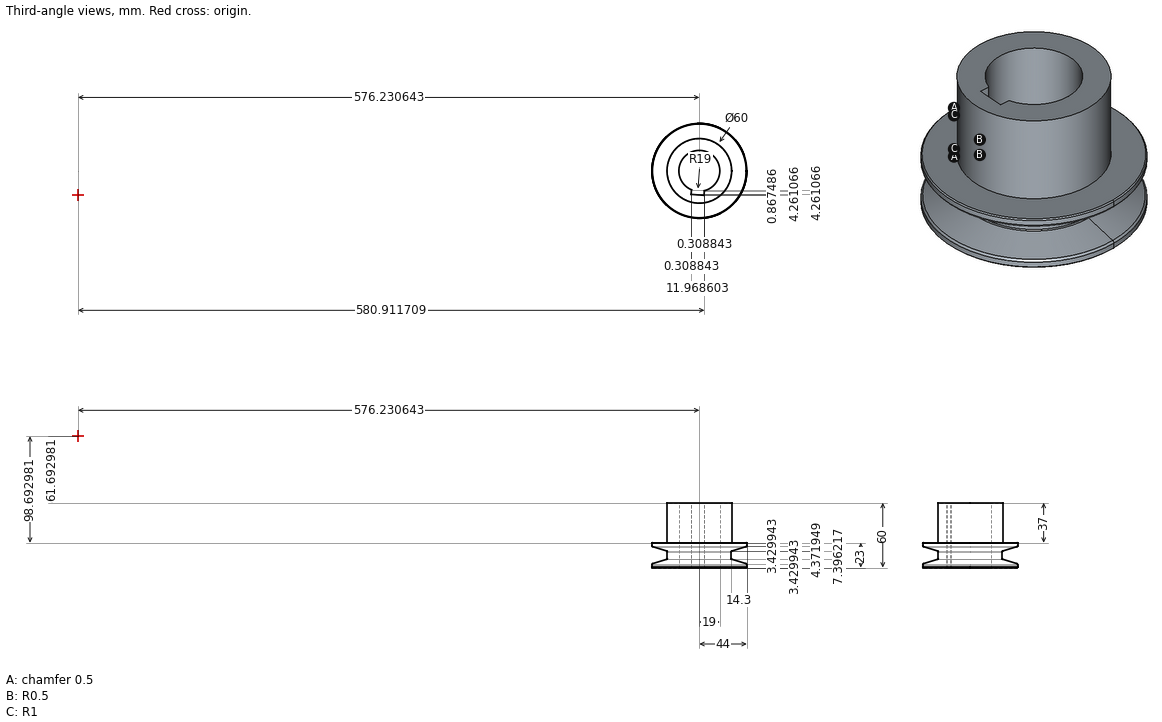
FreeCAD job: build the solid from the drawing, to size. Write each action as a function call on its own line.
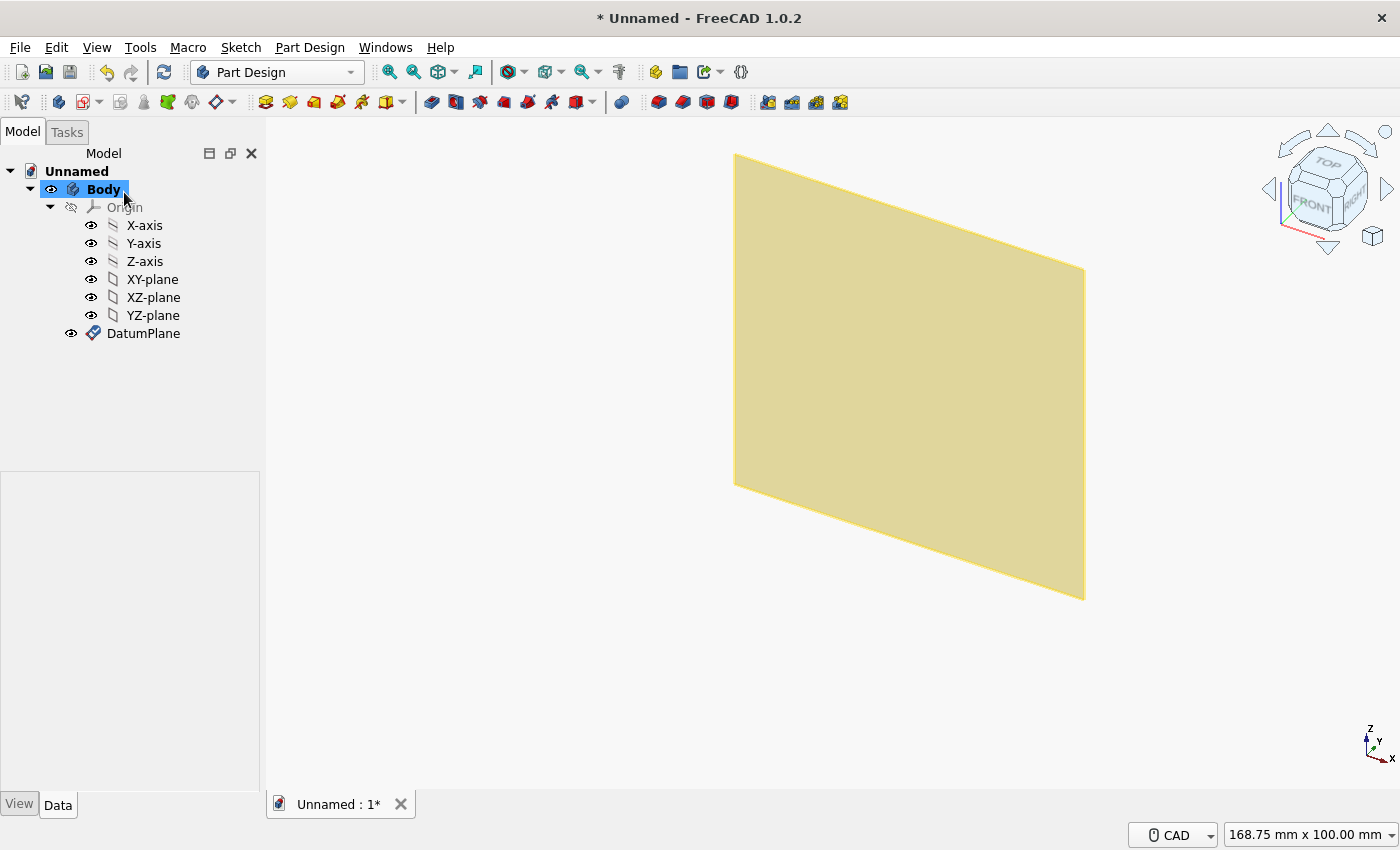
click(116, 333)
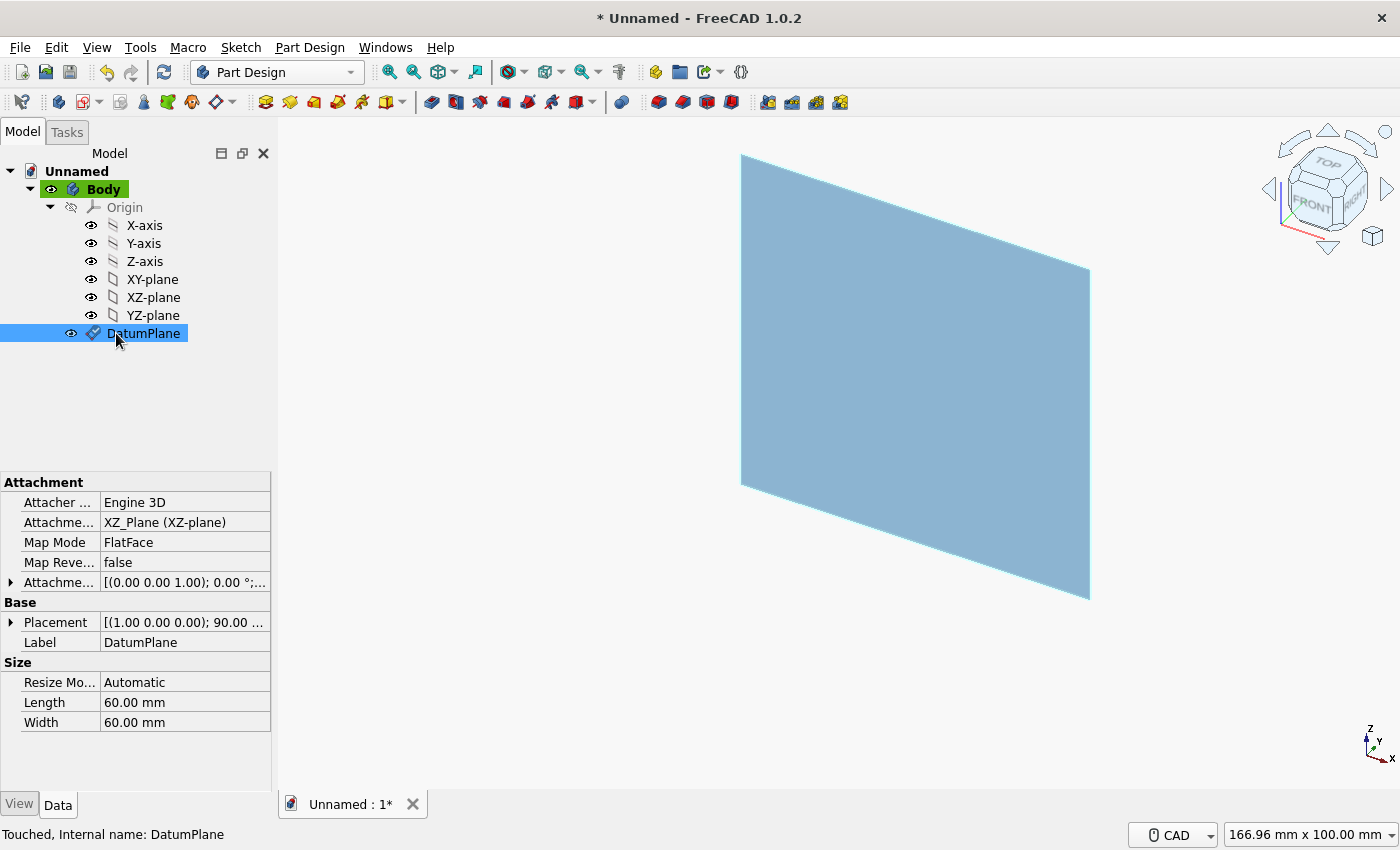
click(84, 102)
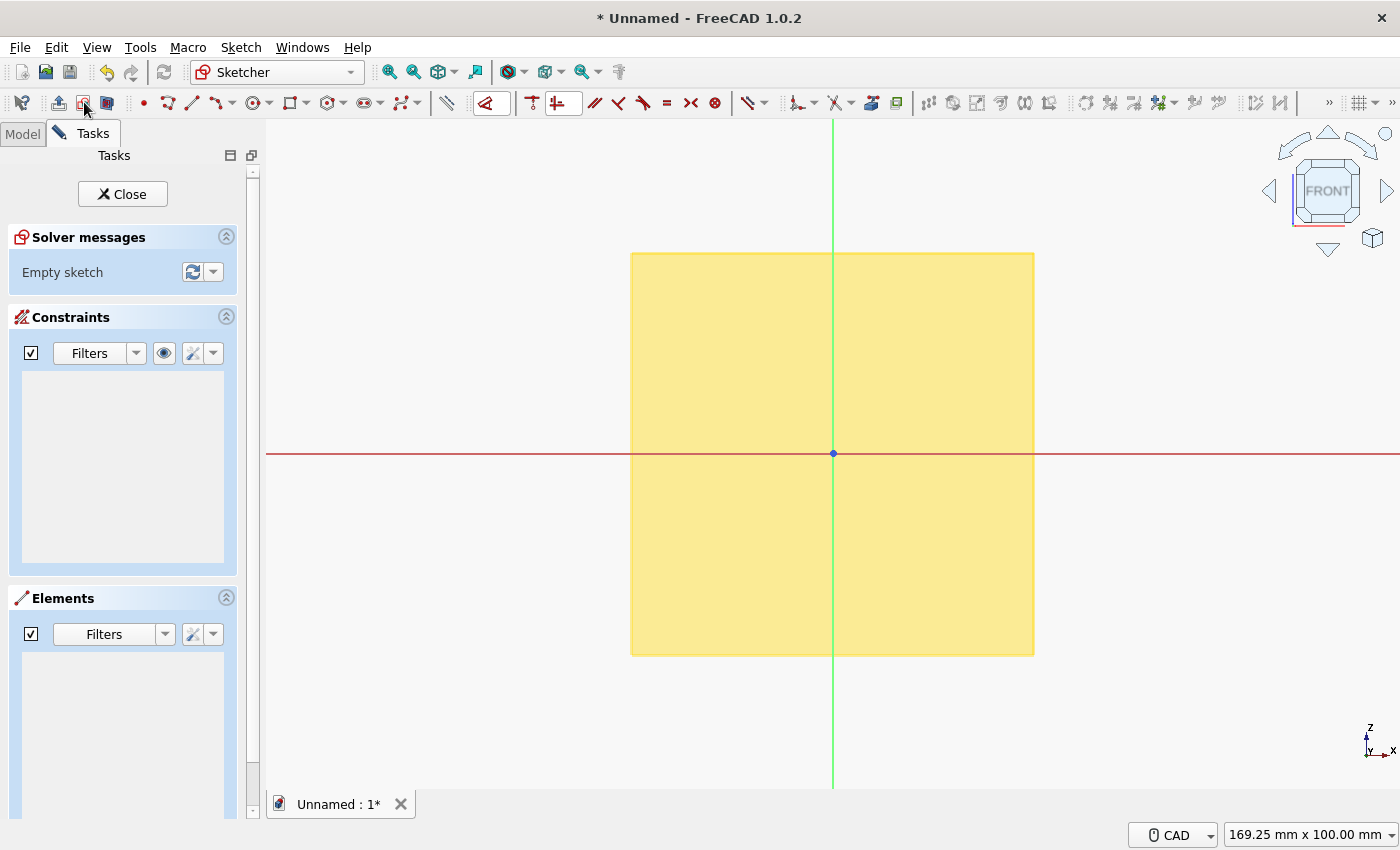
scroll(764, 454, down, 5)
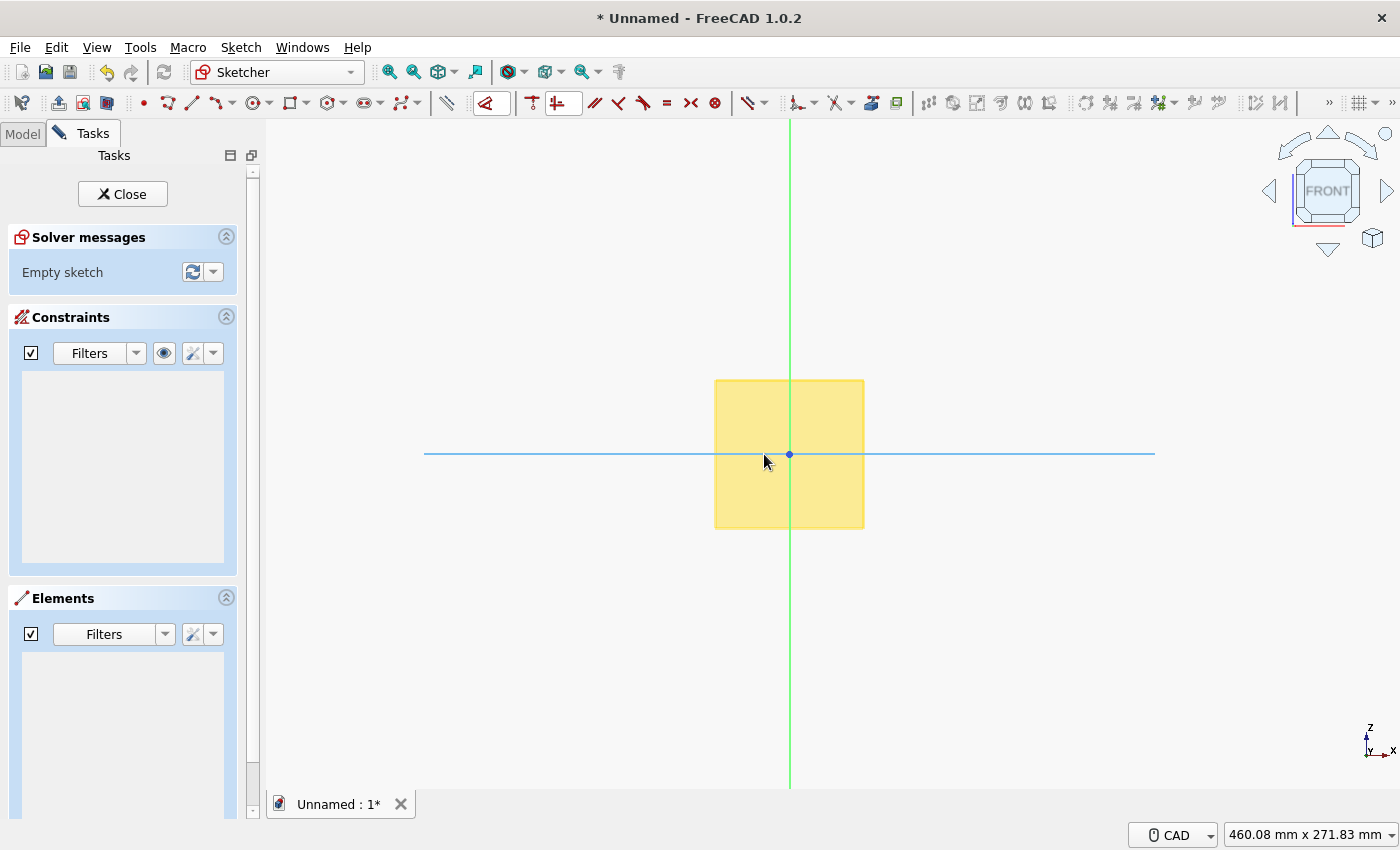
scroll(764, 454, down, 5)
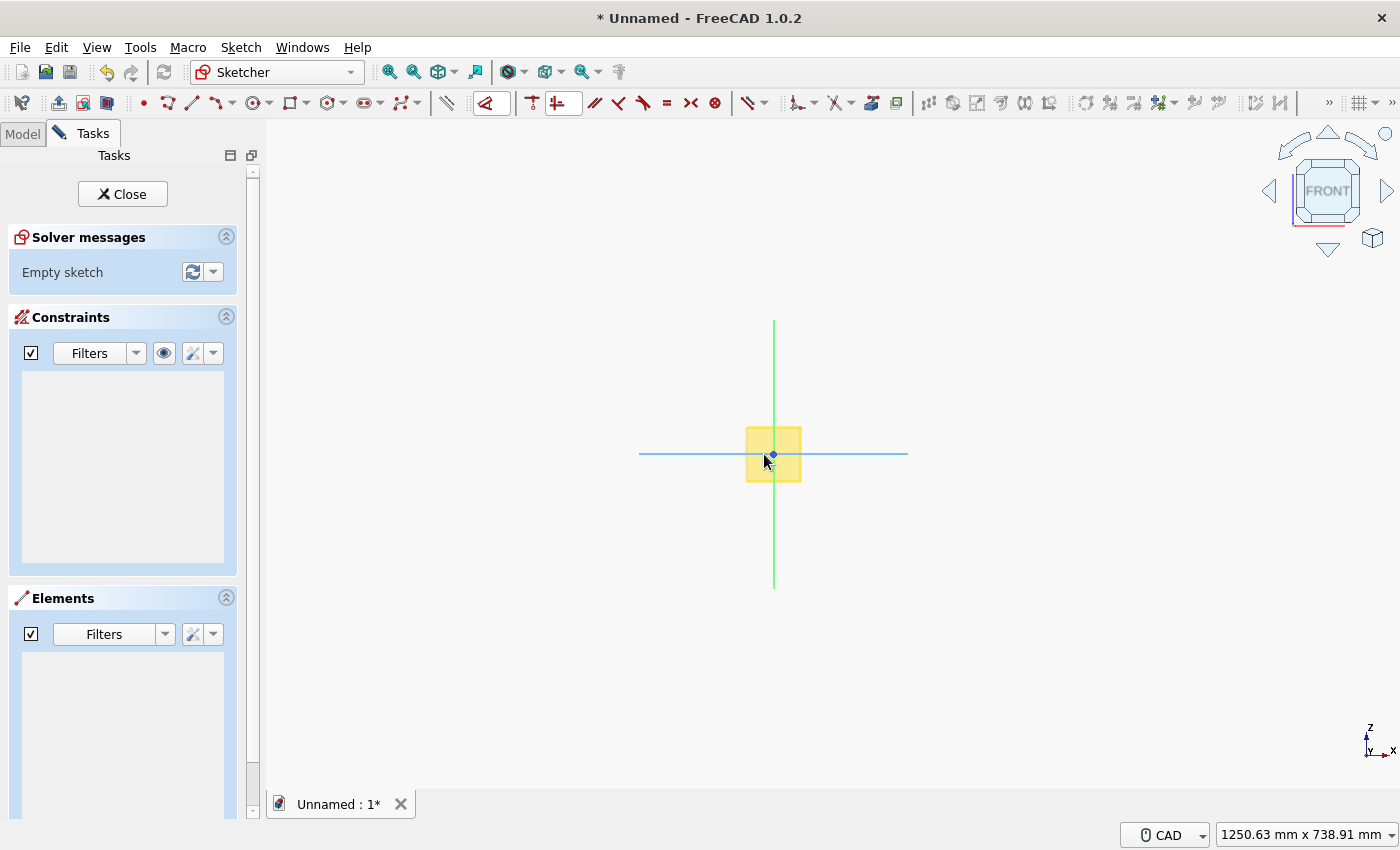
scroll(764, 454, down, 5)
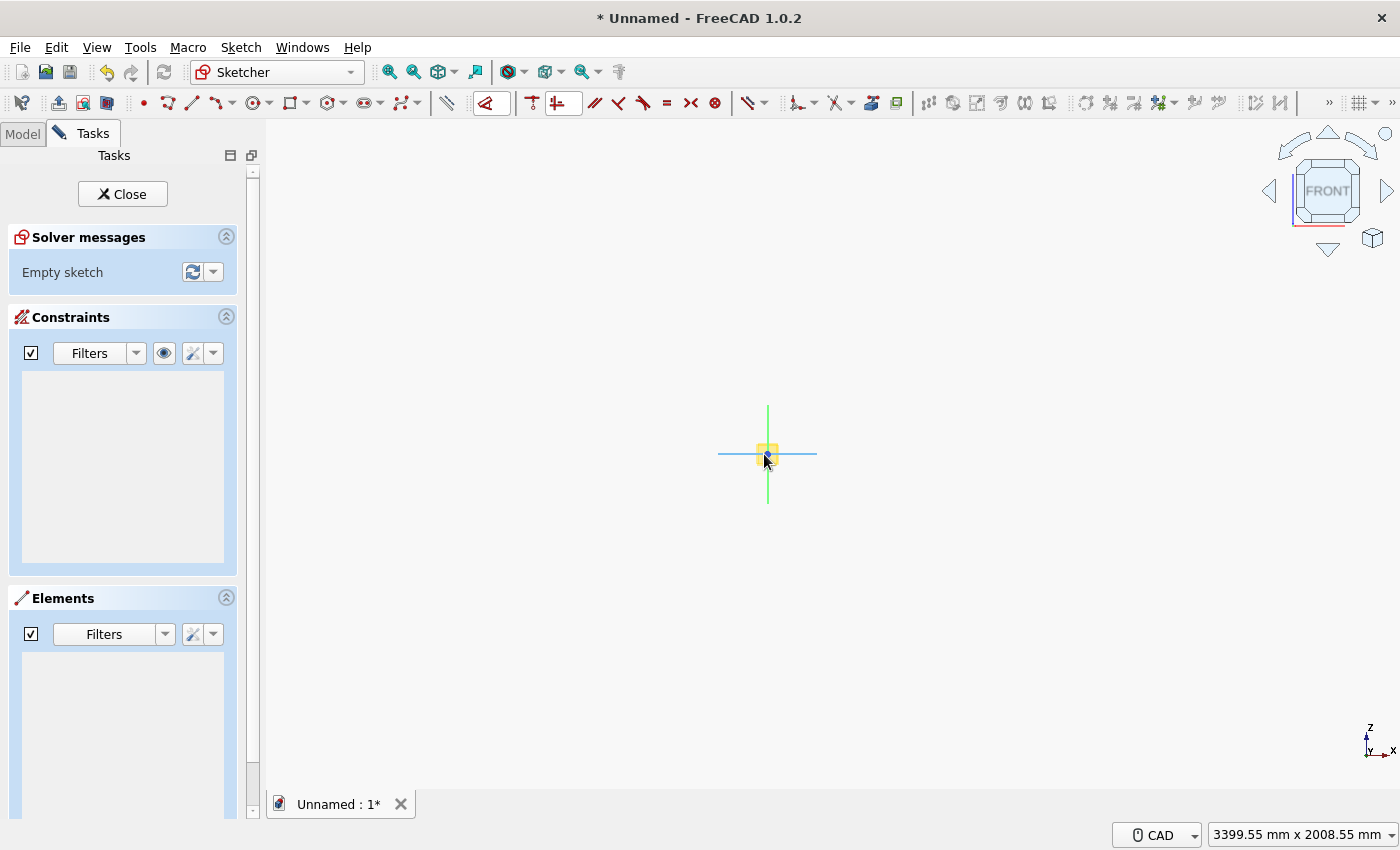
scroll(978, 492, up, 15)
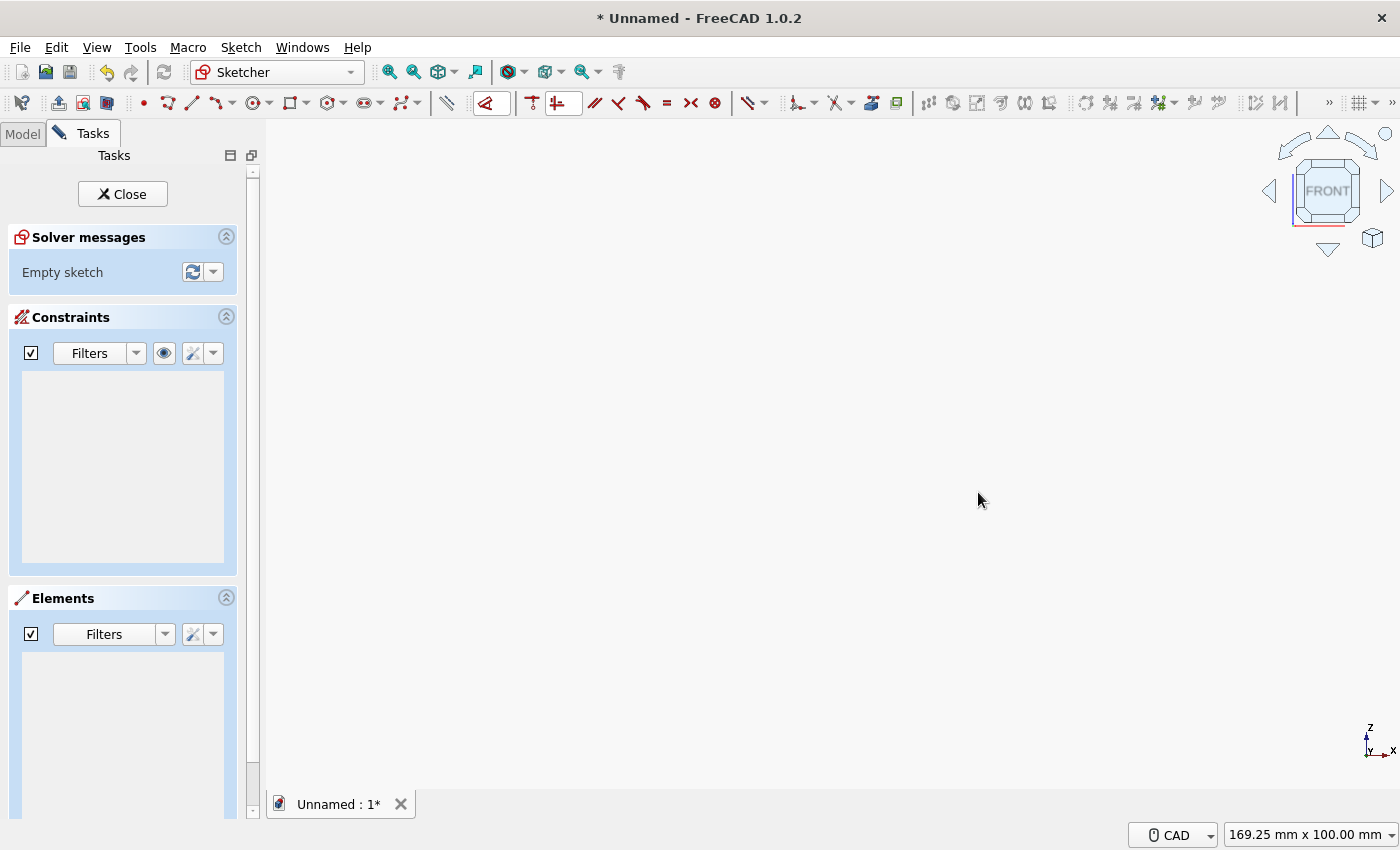
scroll(740, 412, up, 3)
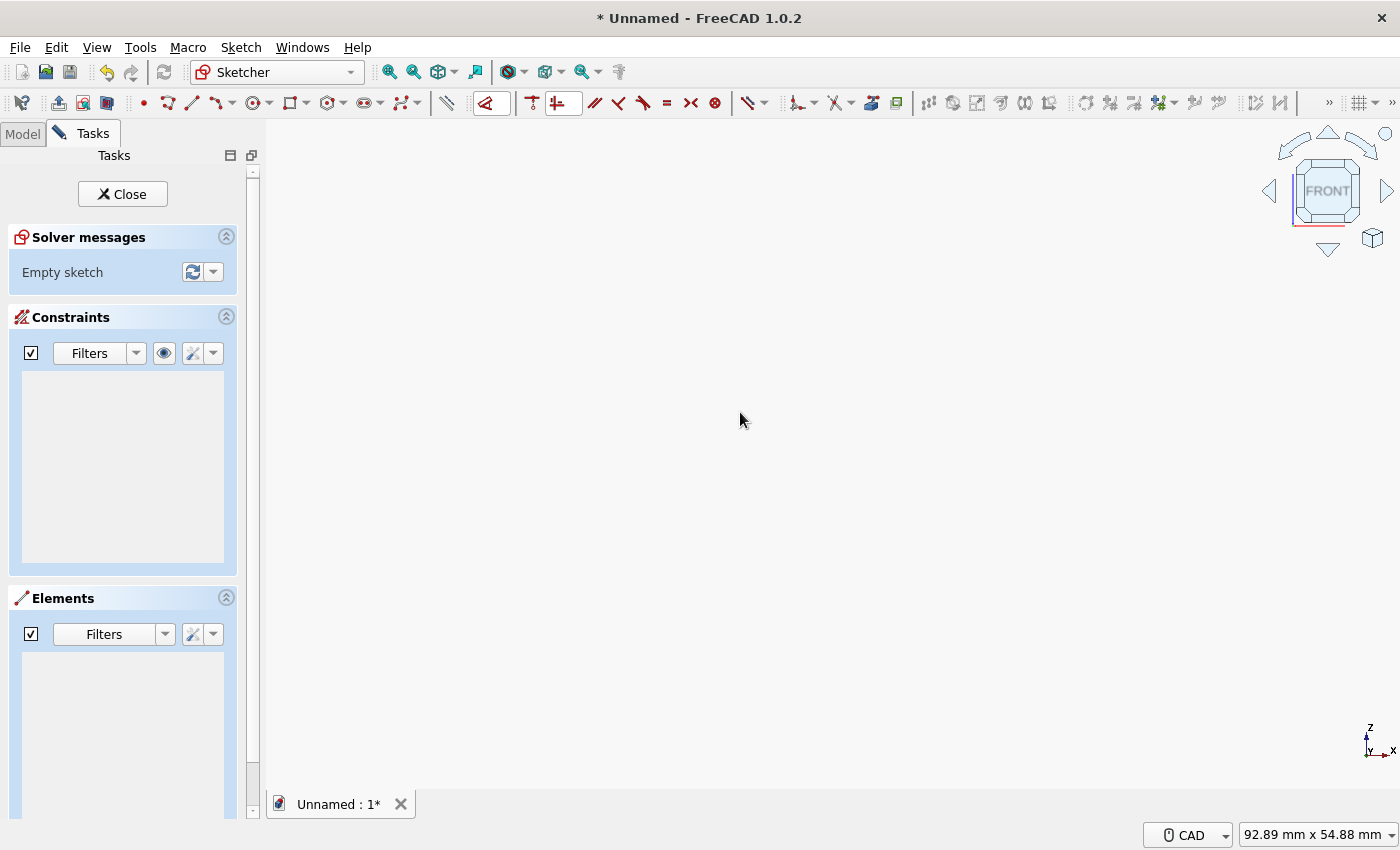
key(g)
key(m)